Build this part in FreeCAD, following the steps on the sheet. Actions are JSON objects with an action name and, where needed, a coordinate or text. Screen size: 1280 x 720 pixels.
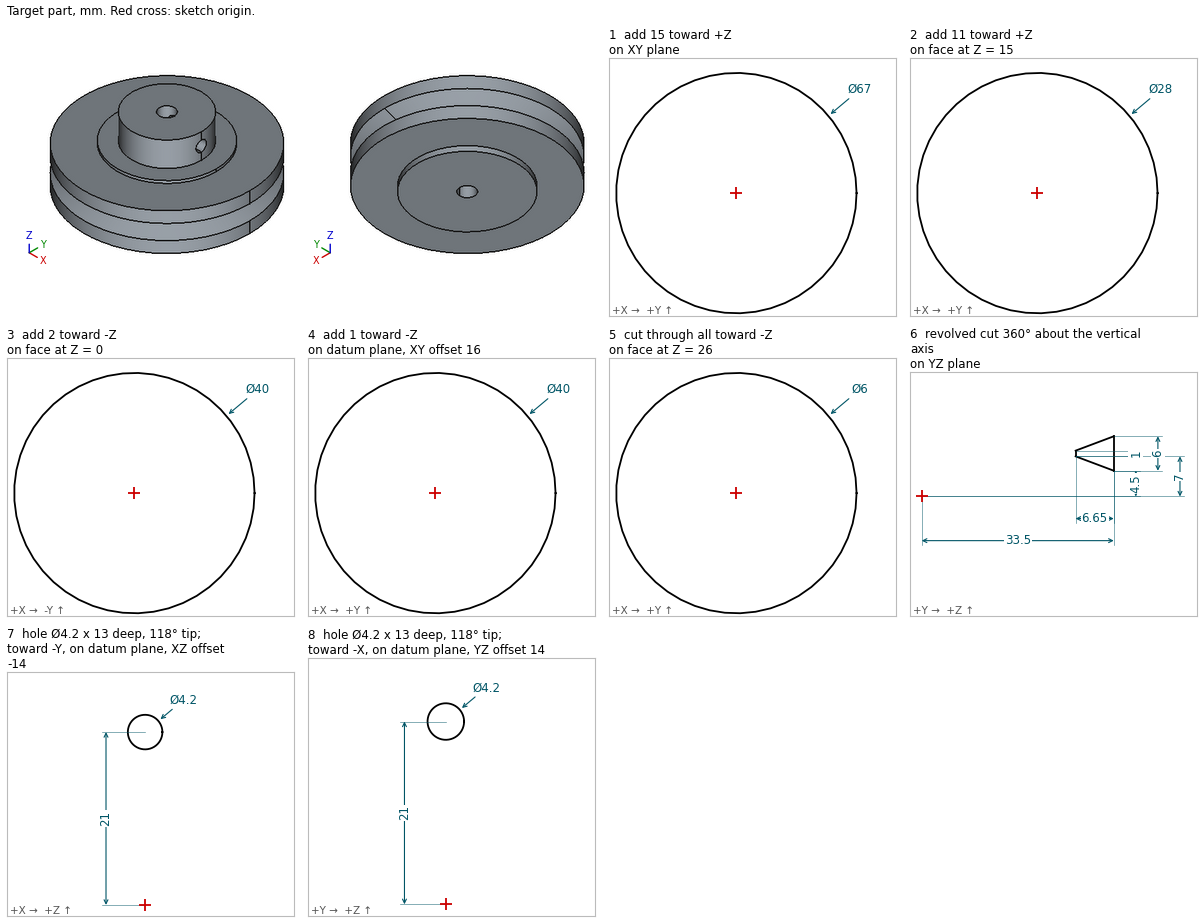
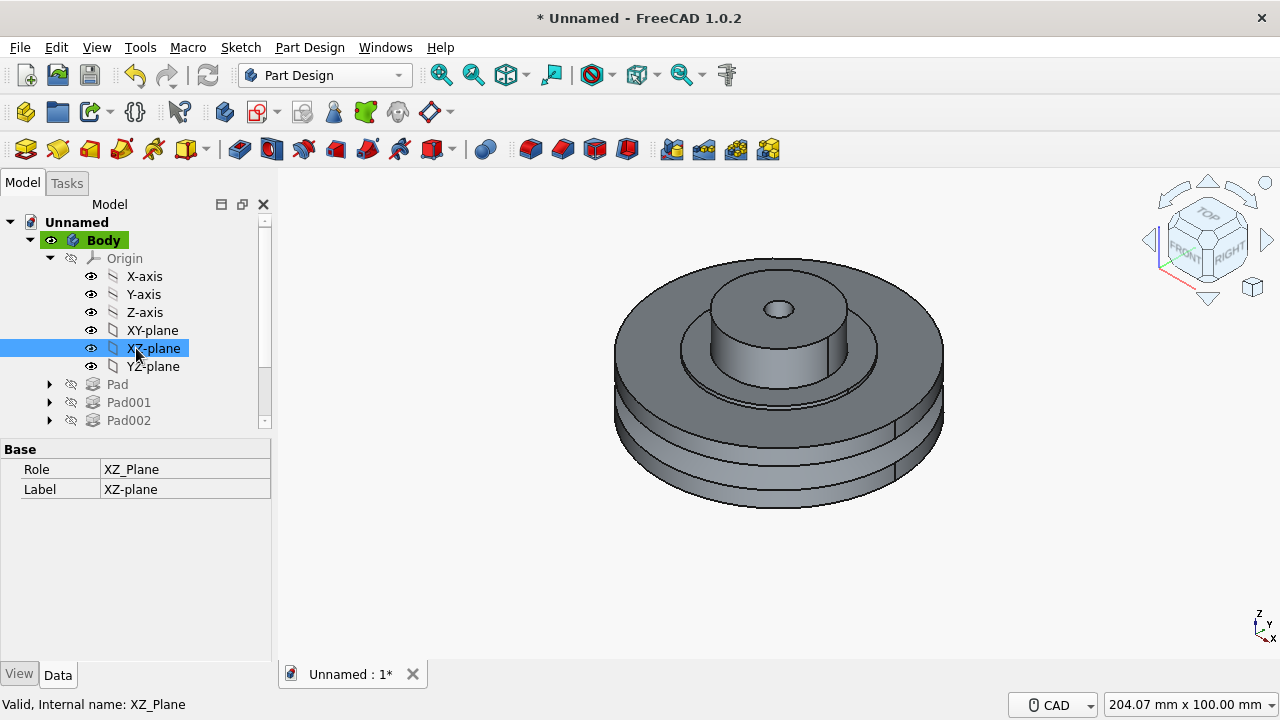
{"action": "left_click", "coordinate": [430, 112]}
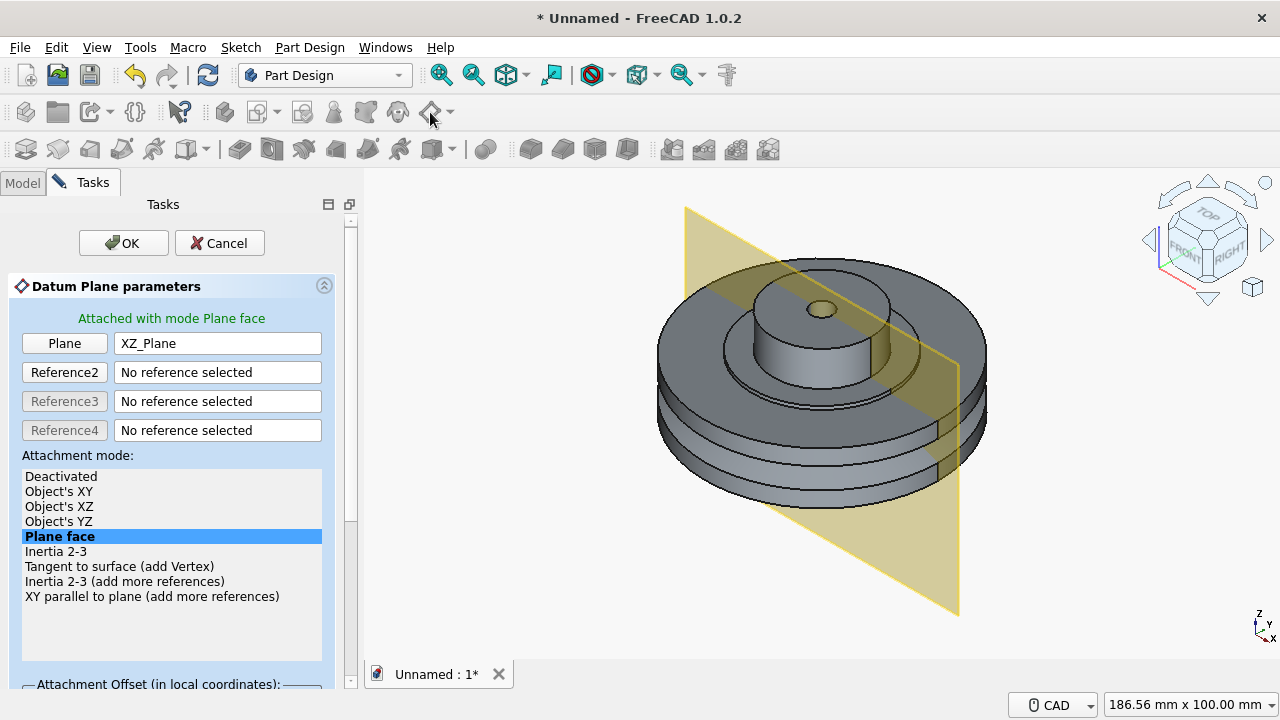
{"action": "scroll", "coordinate": [351, 451], "scroll_direction": "down", "scroll_amount": 3}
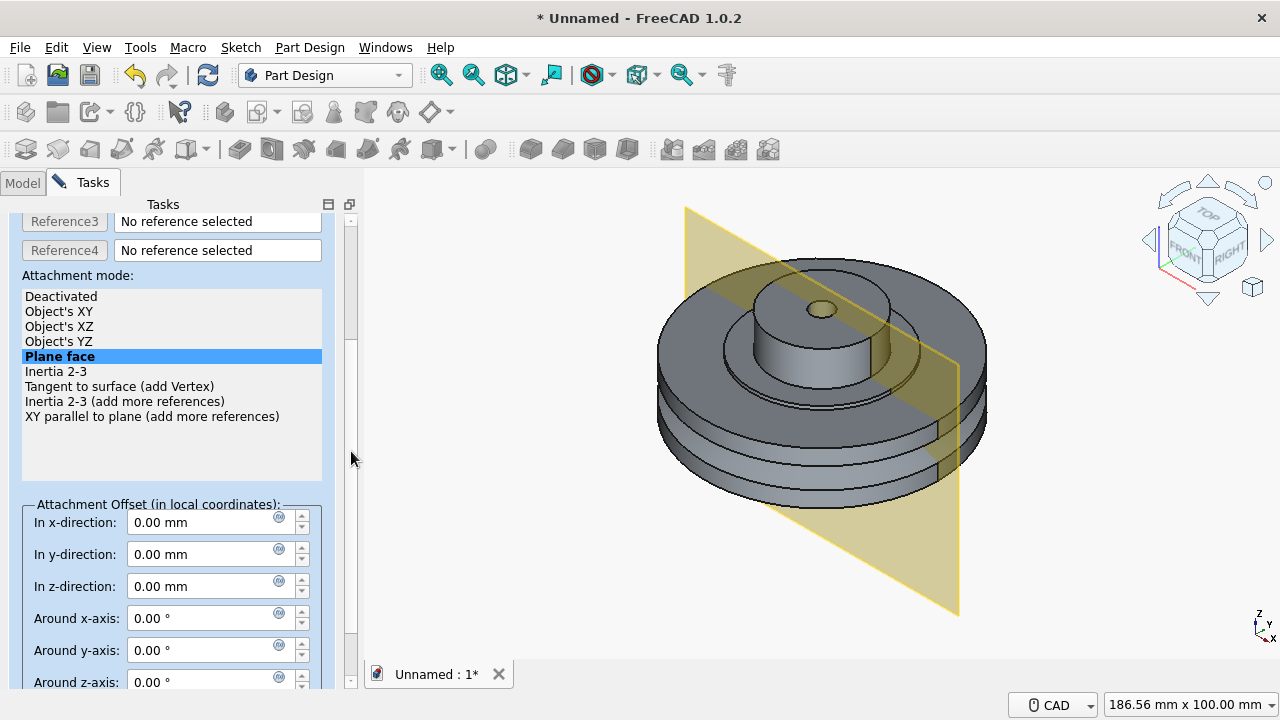
{"action": "triple_click", "coordinate": [210, 586]}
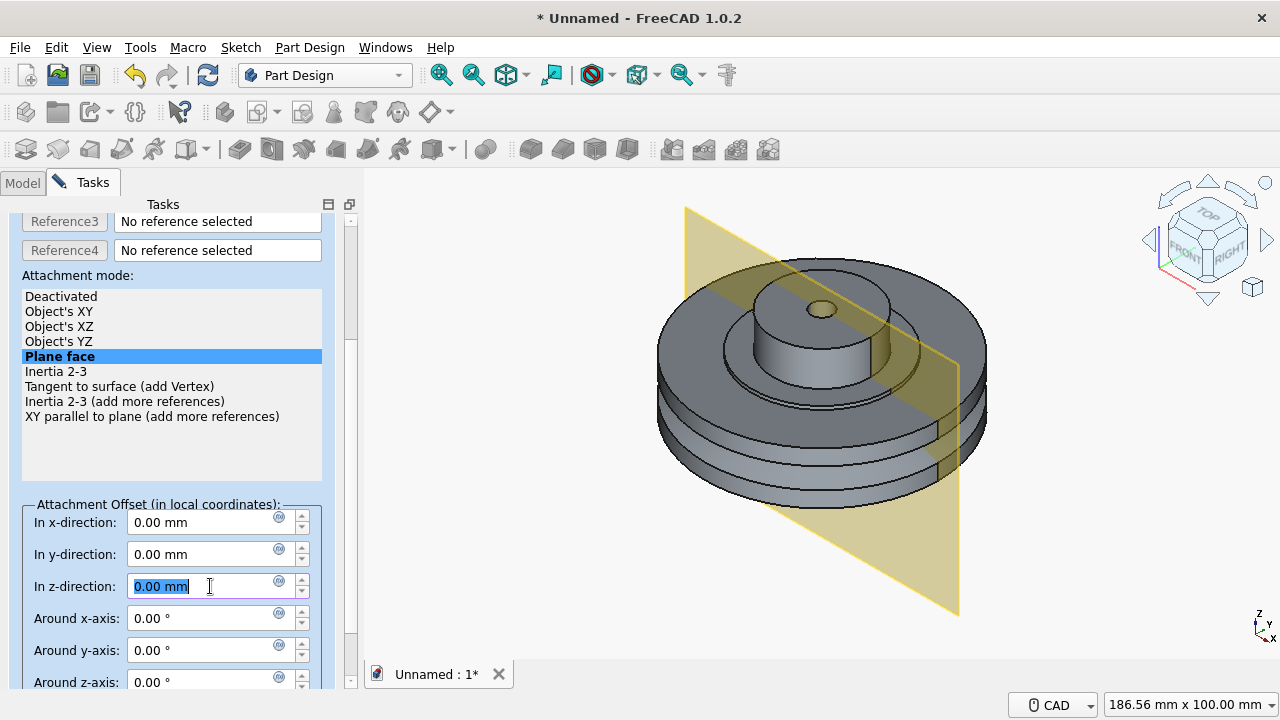
{"action": "type", "text": "-14"}
{"action": "key", "text": "Tab"}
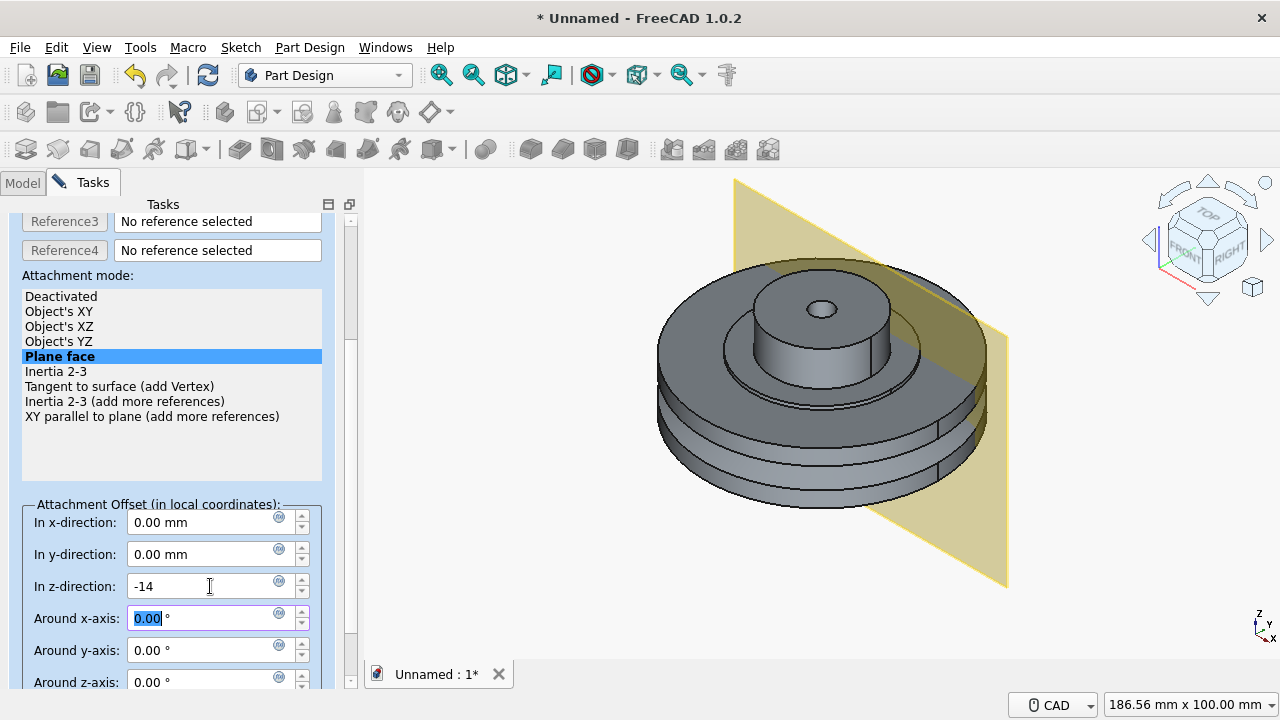
{"action": "scroll", "coordinate": [351, 451], "scroll_direction": "up", "scroll_amount": 4}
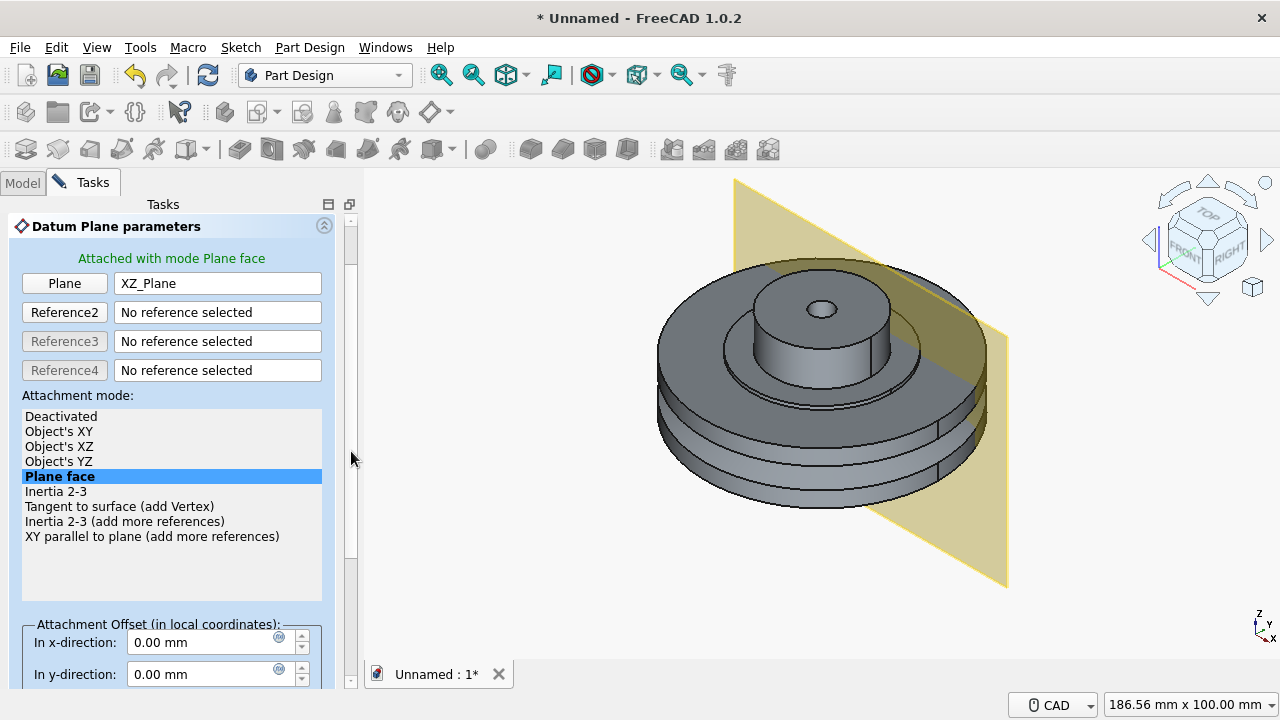
{"action": "left_click", "coordinate": [124, 243]}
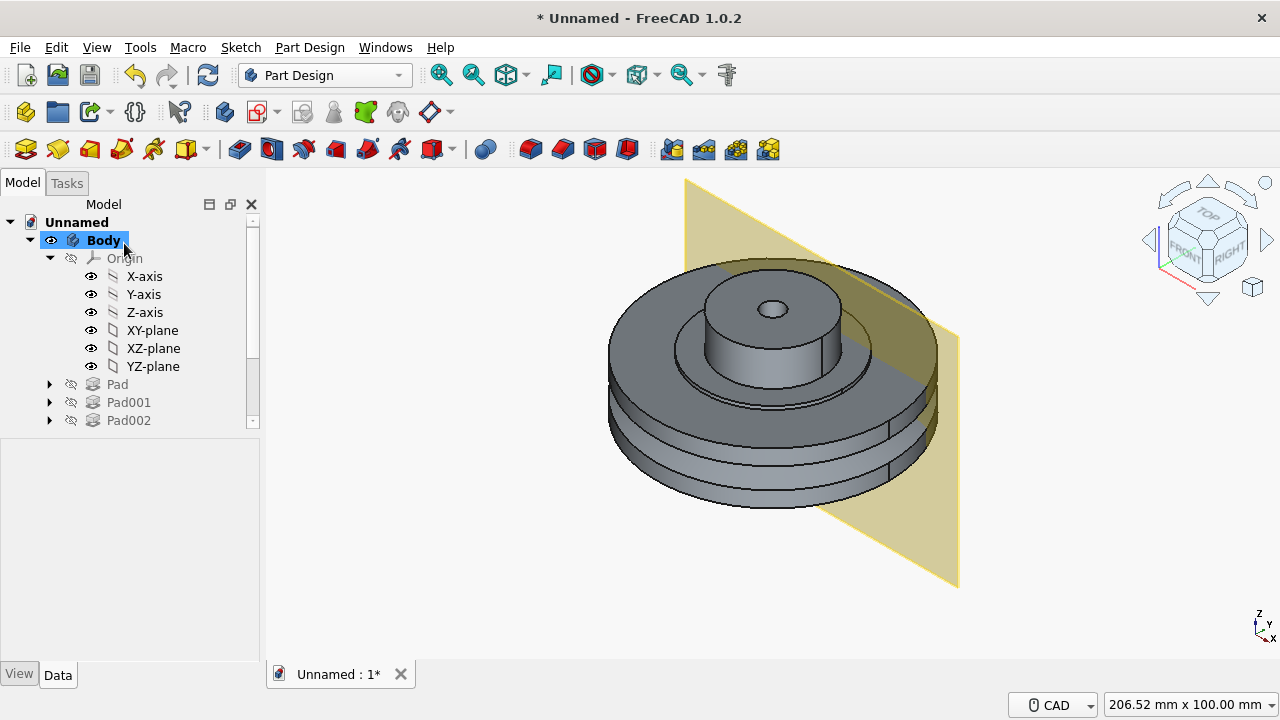
{"action": "scroll", "coordinate": [100, 326], "scroll_direction": "down", "scroll_amount": 3}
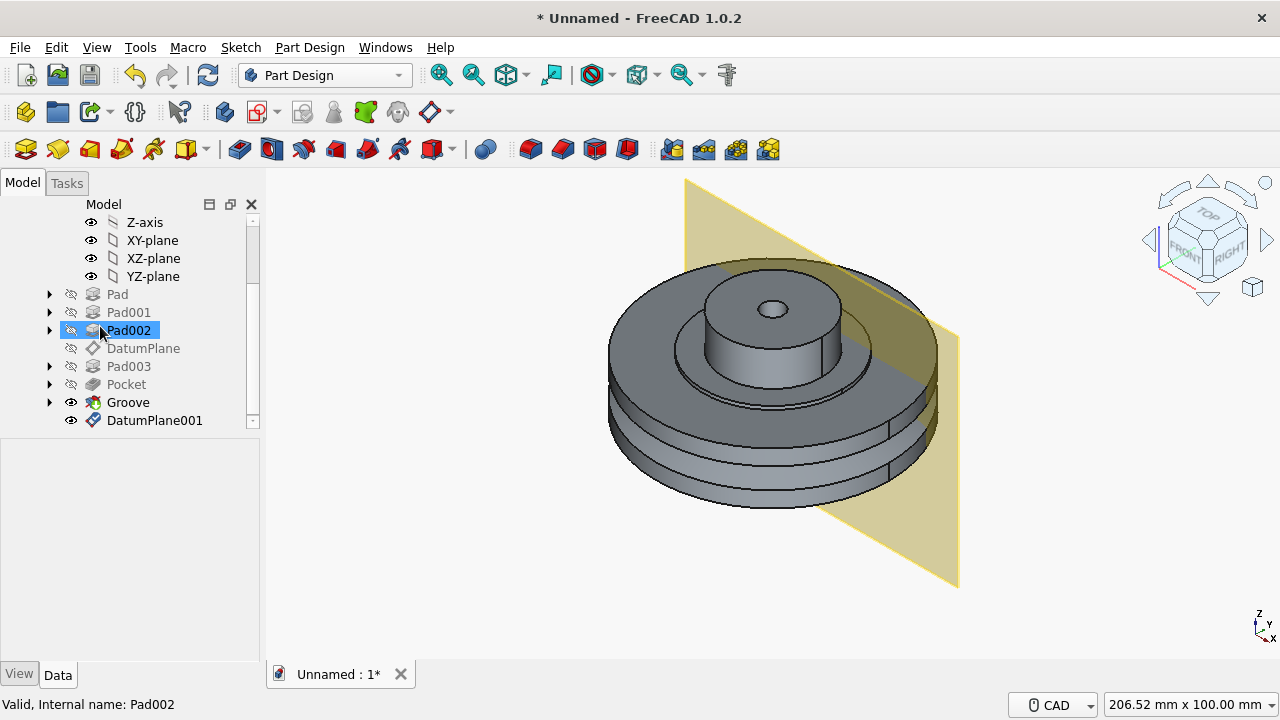
{"action": "left_click", "coordinate": [116, 420]}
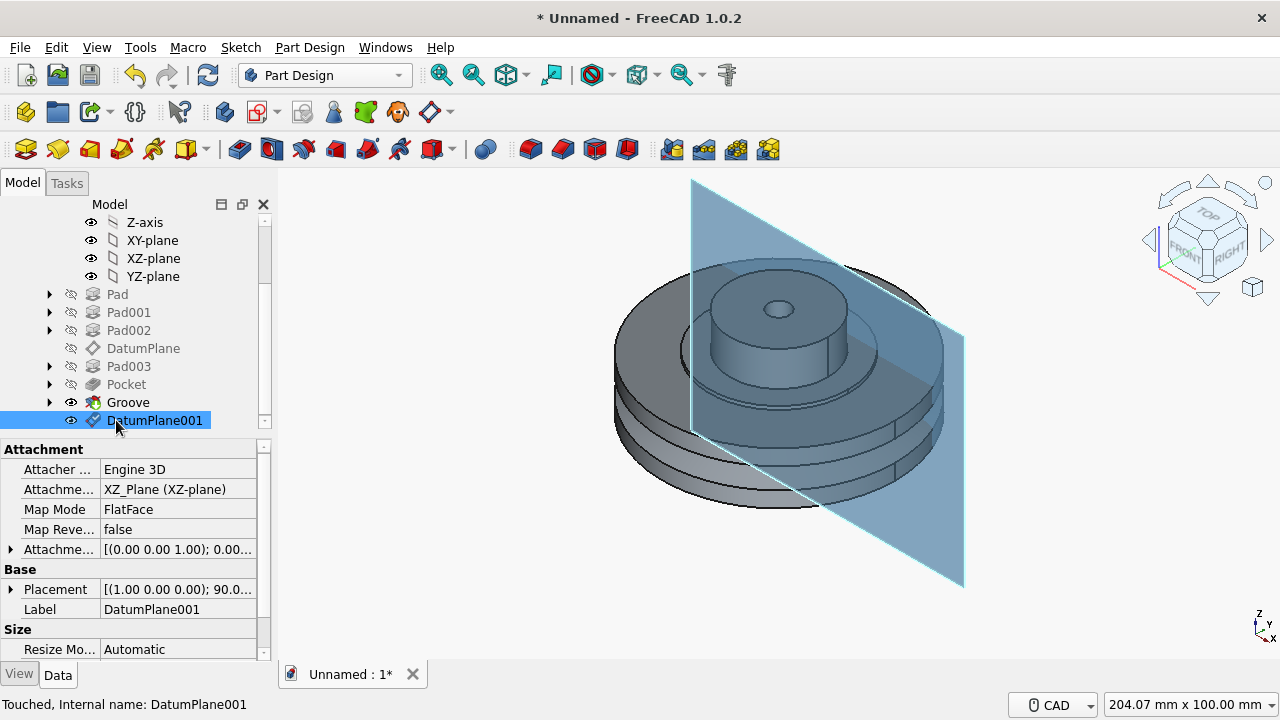
{"action": "left_click", "coordinate": [258, 112]}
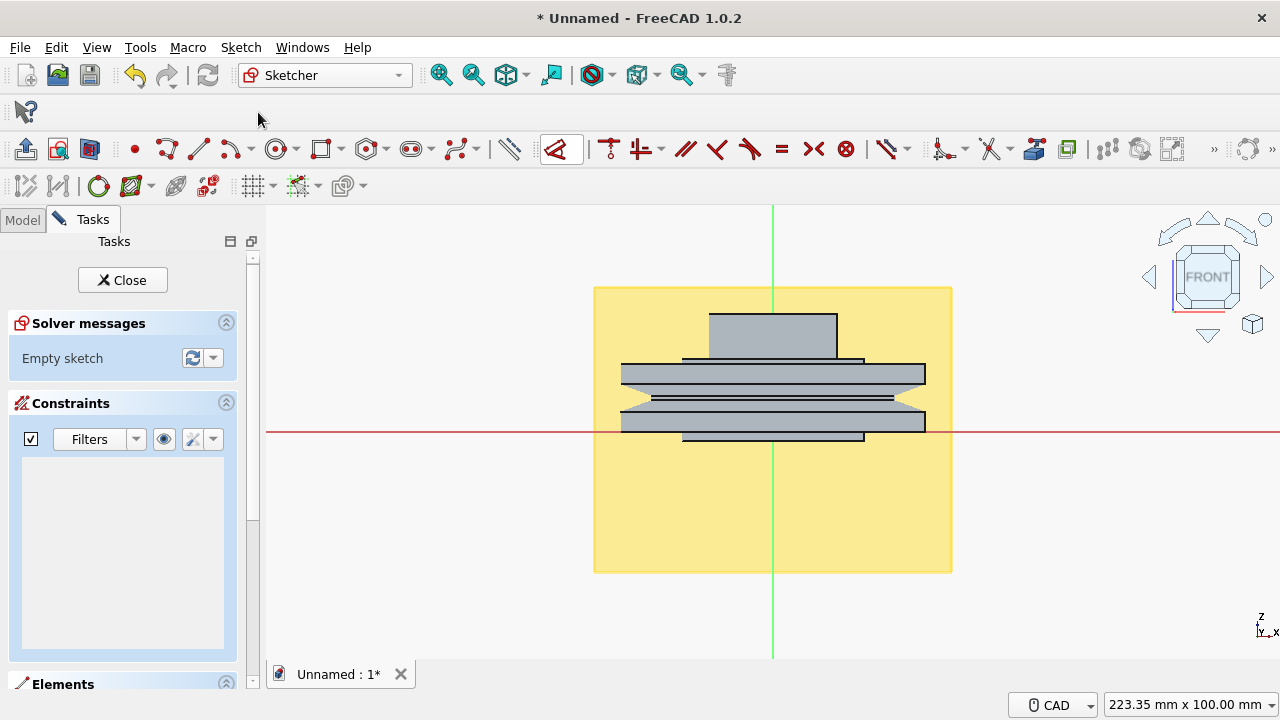
{"action": "left_click", "coordinate": [90, 150]}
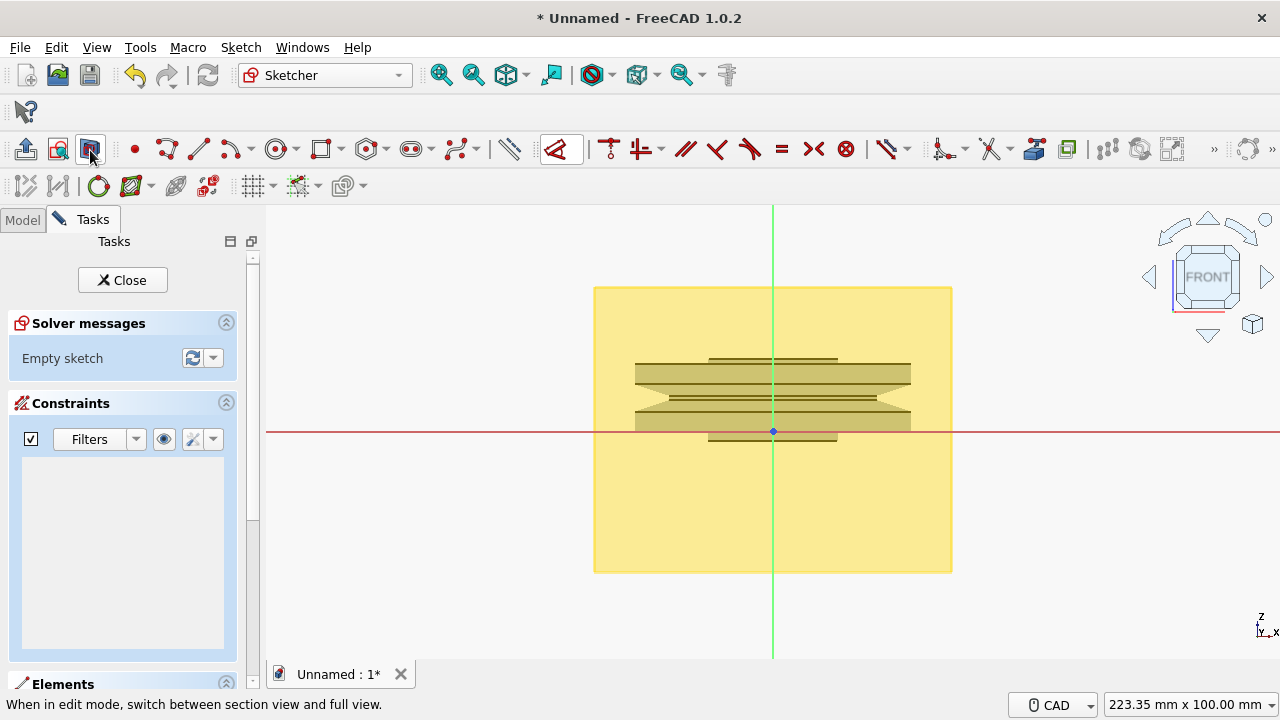
{"action": "scroll", "coordinate": [778, 329], "scroll_direction": "up", "scroll_amount": 13}